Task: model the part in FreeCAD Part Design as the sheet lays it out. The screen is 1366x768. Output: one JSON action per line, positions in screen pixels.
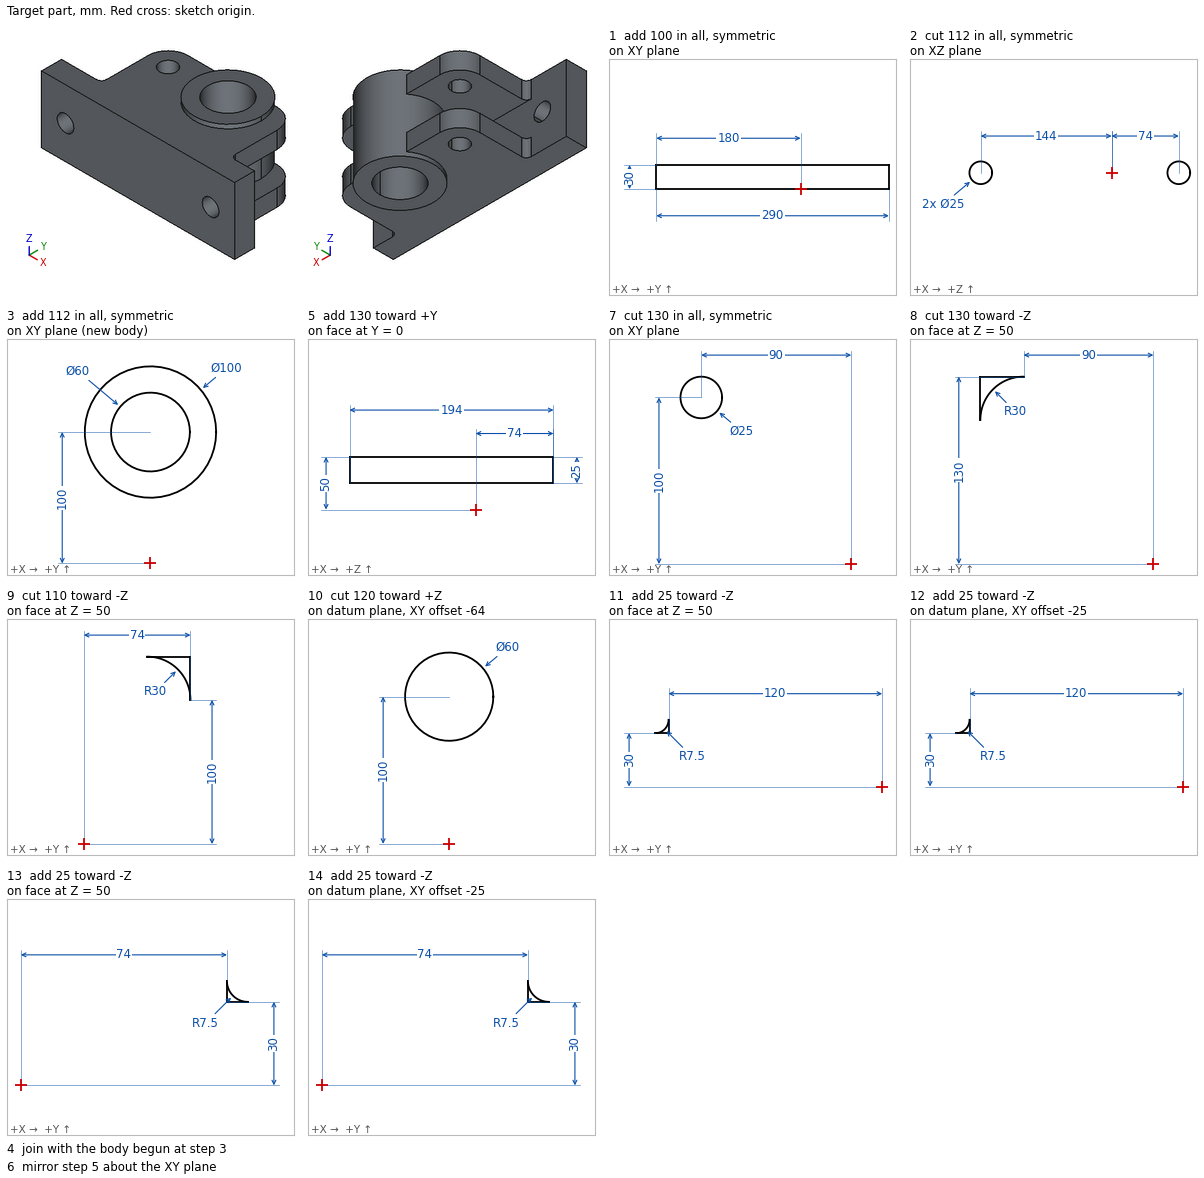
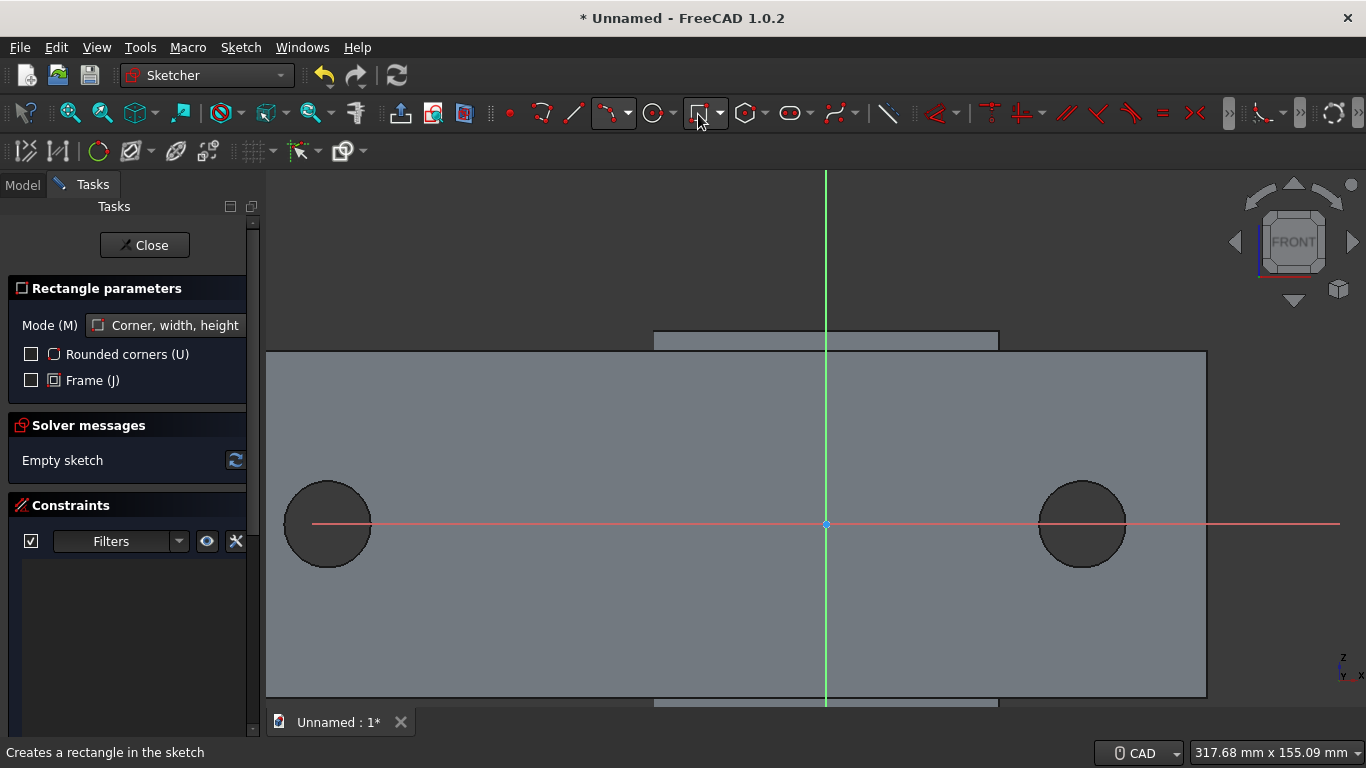
{"action": "left_click", "coordinate": [411, 351]}
{"action": "mouse_move", "coordinate": [1082, 438]}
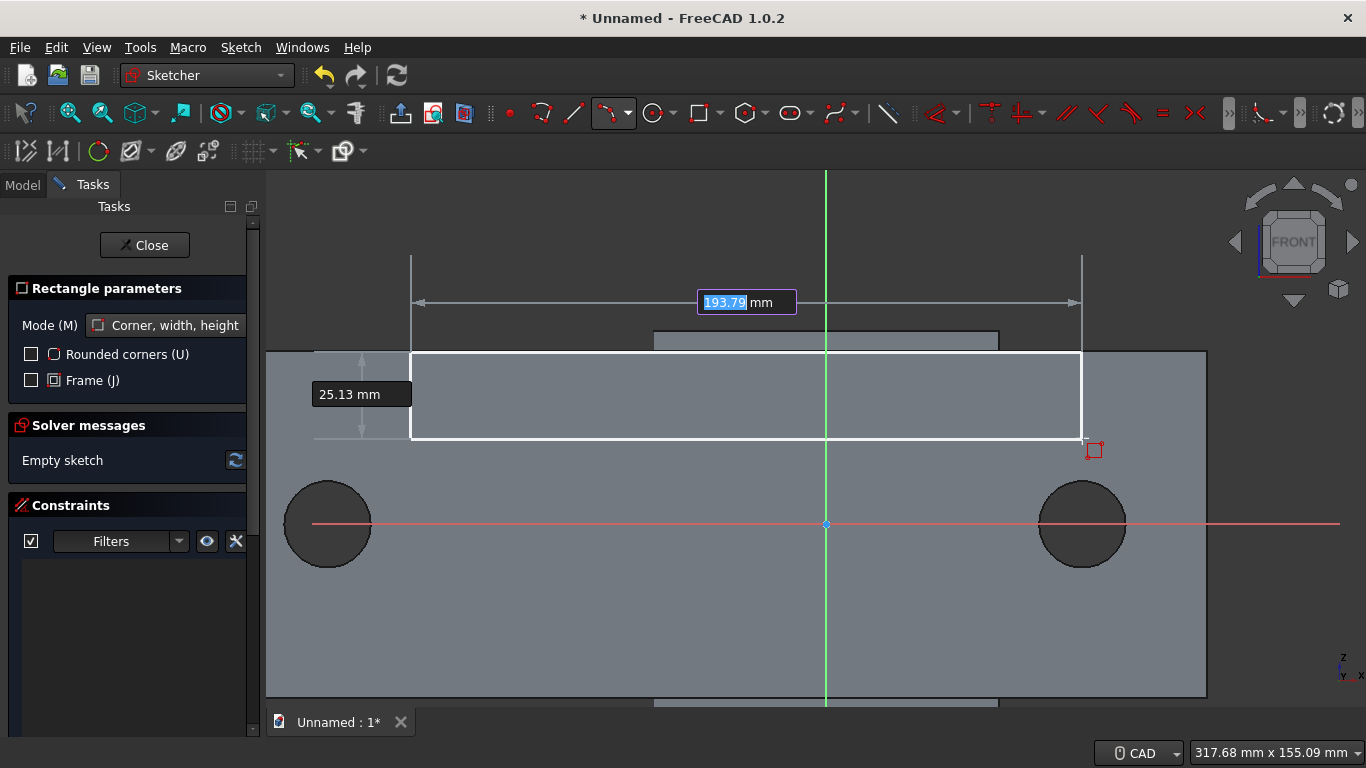
{"action": "type", "text": "194"}
{"action": "key", "text": "Tab"}
{"action": "type", "text": "25"}
{"action": "key", "text": "Return"}
{"action": "key", "text": "Escape"}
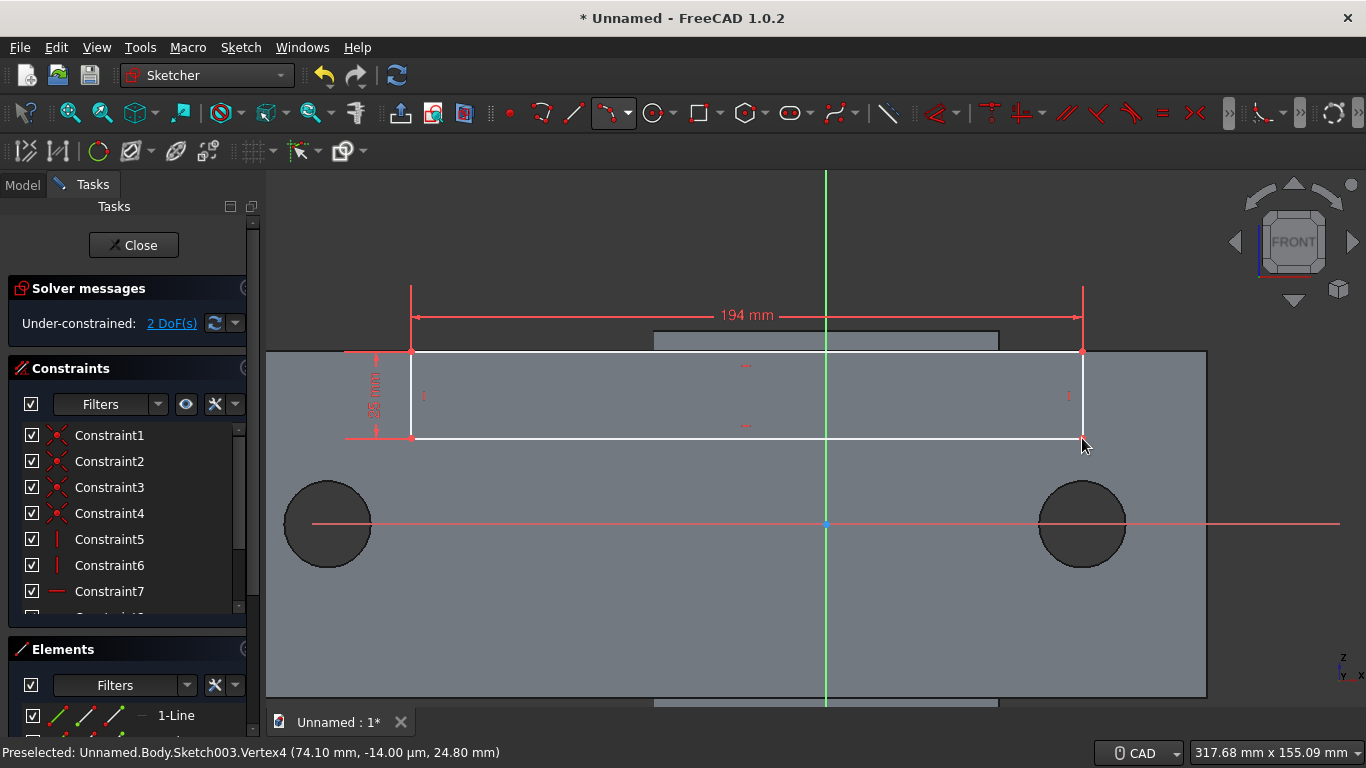
{"action": "left_click", "coordinate": [936, 114]}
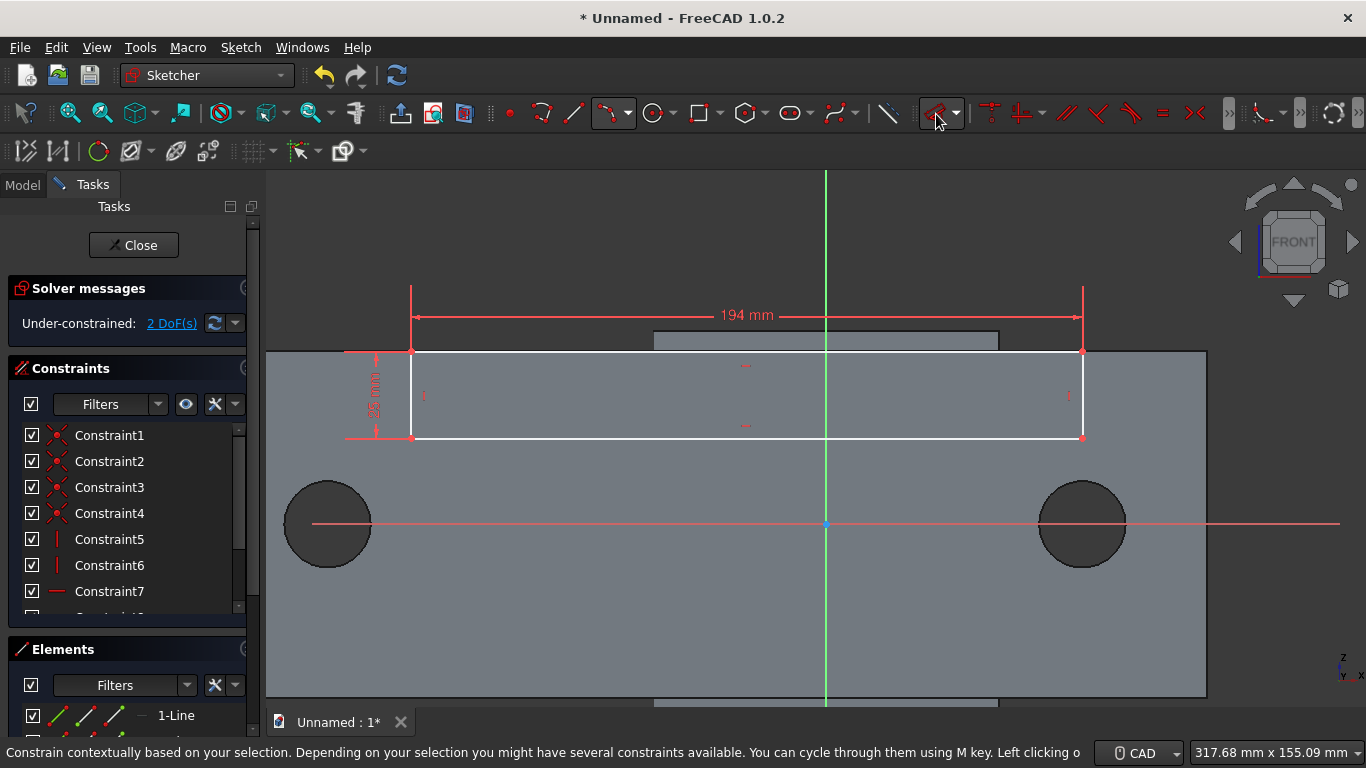
{"action": "left_click", "coordinate": [411, 352]}
{"action": "left_click", "coordinate": [377, 438]}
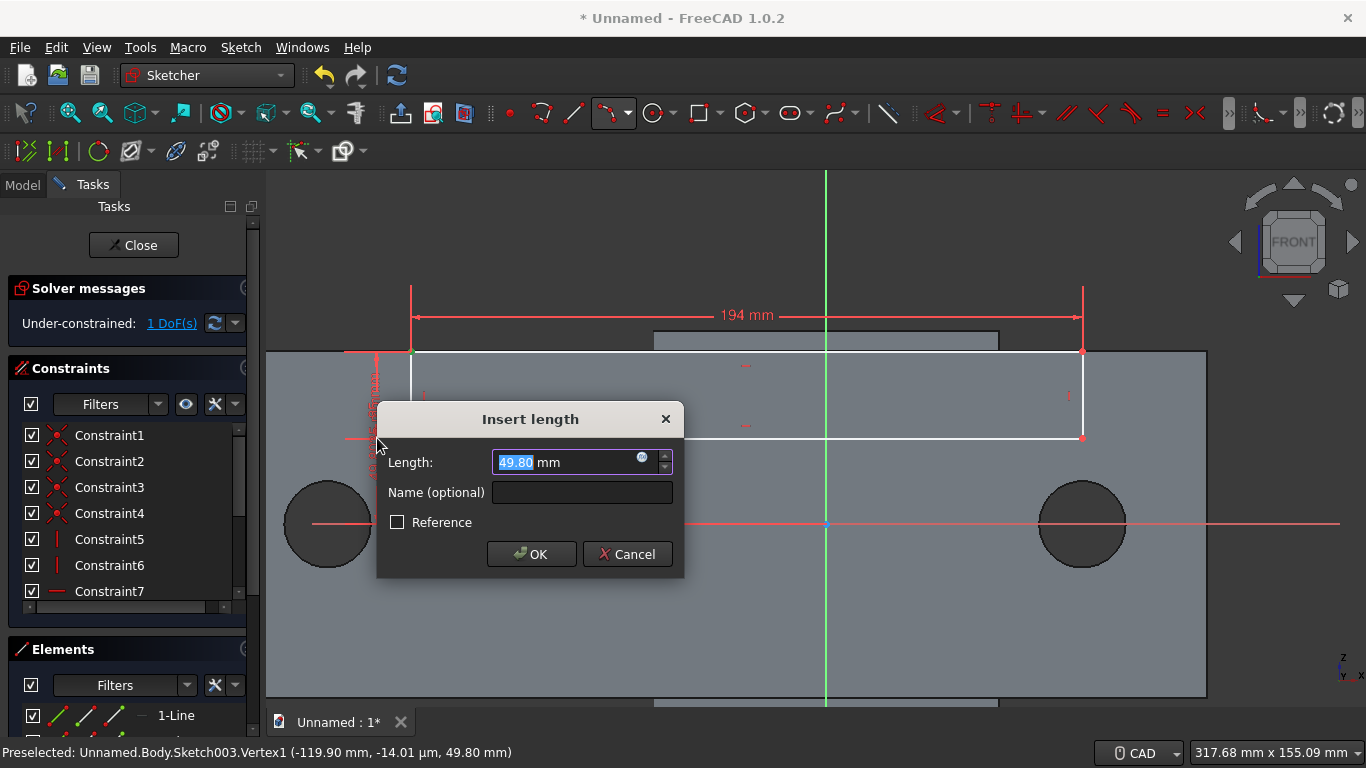
{"action": "type", "text": "50"}
{"action": "key", "text": "Return"}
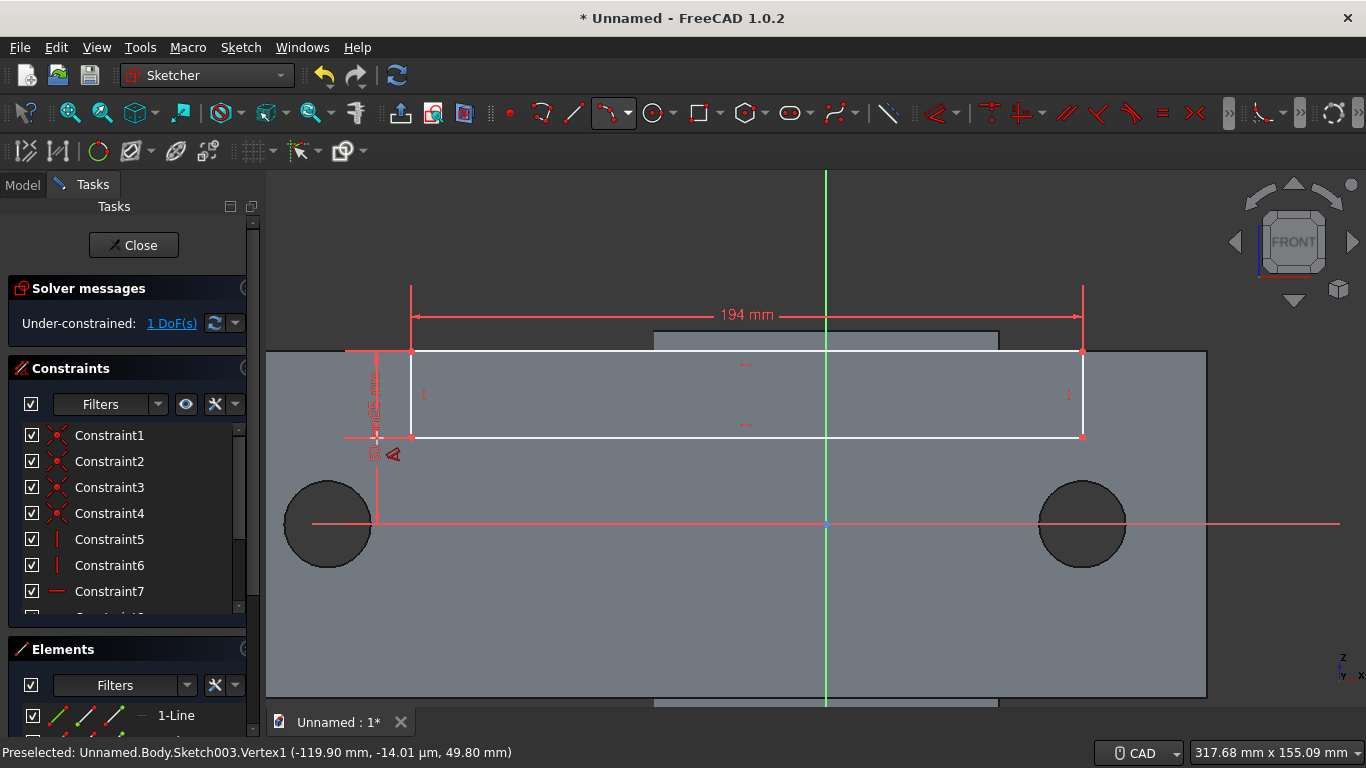
{"action": "left_click", "coordinate": [1083, 438]}
{"action": "left_click", "coordinate": [954, 558]}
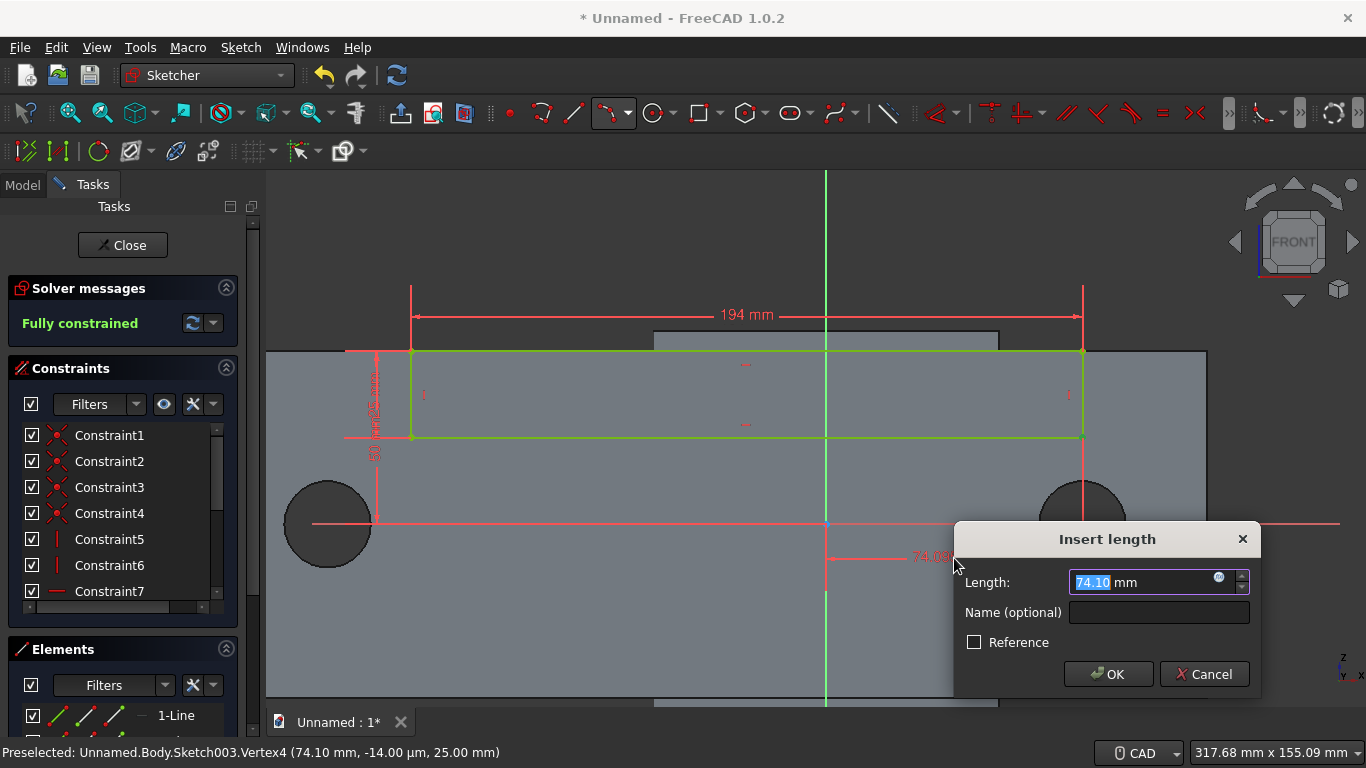
{"action": "type", "text": "74"}
{"action": "key", "text": "Return"}
{"action": "key", "text": "Escape"}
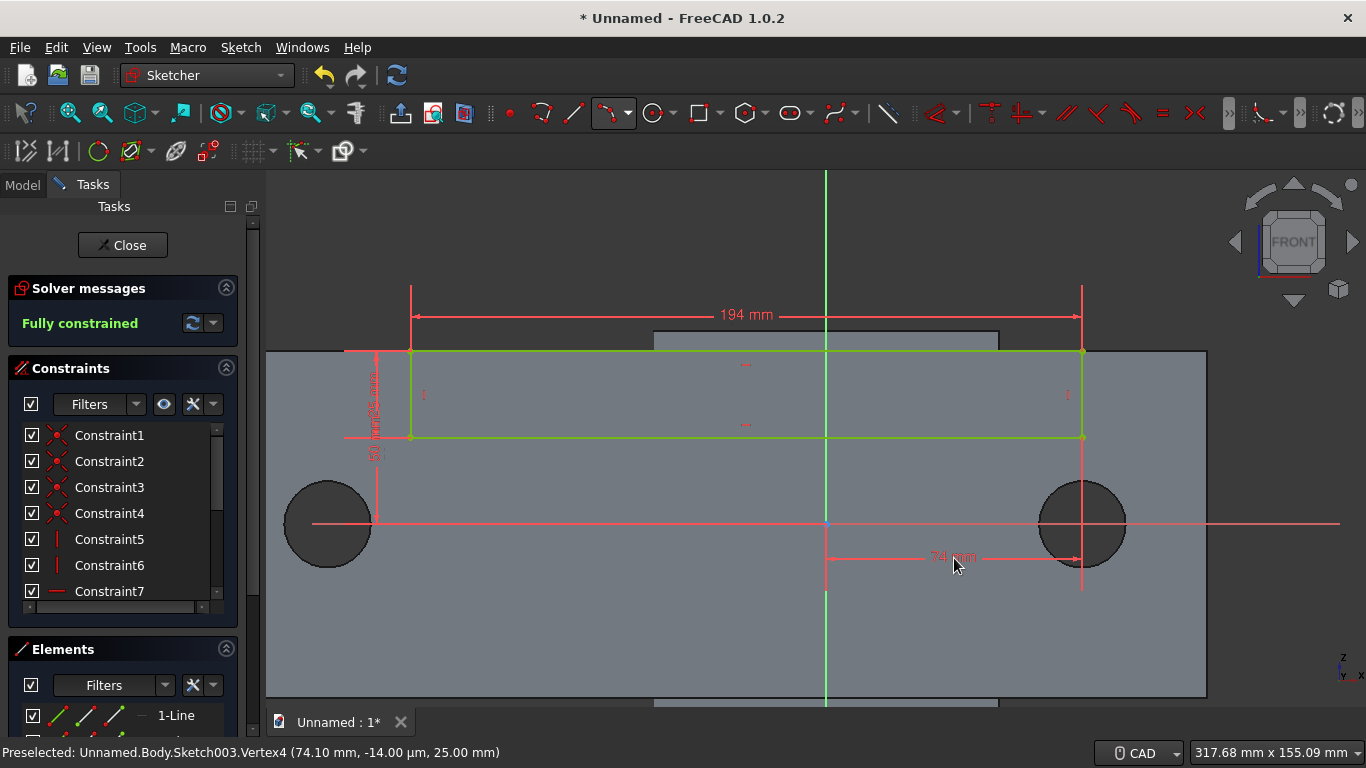
{"action": "left_click", "coordinate": [123, 245]}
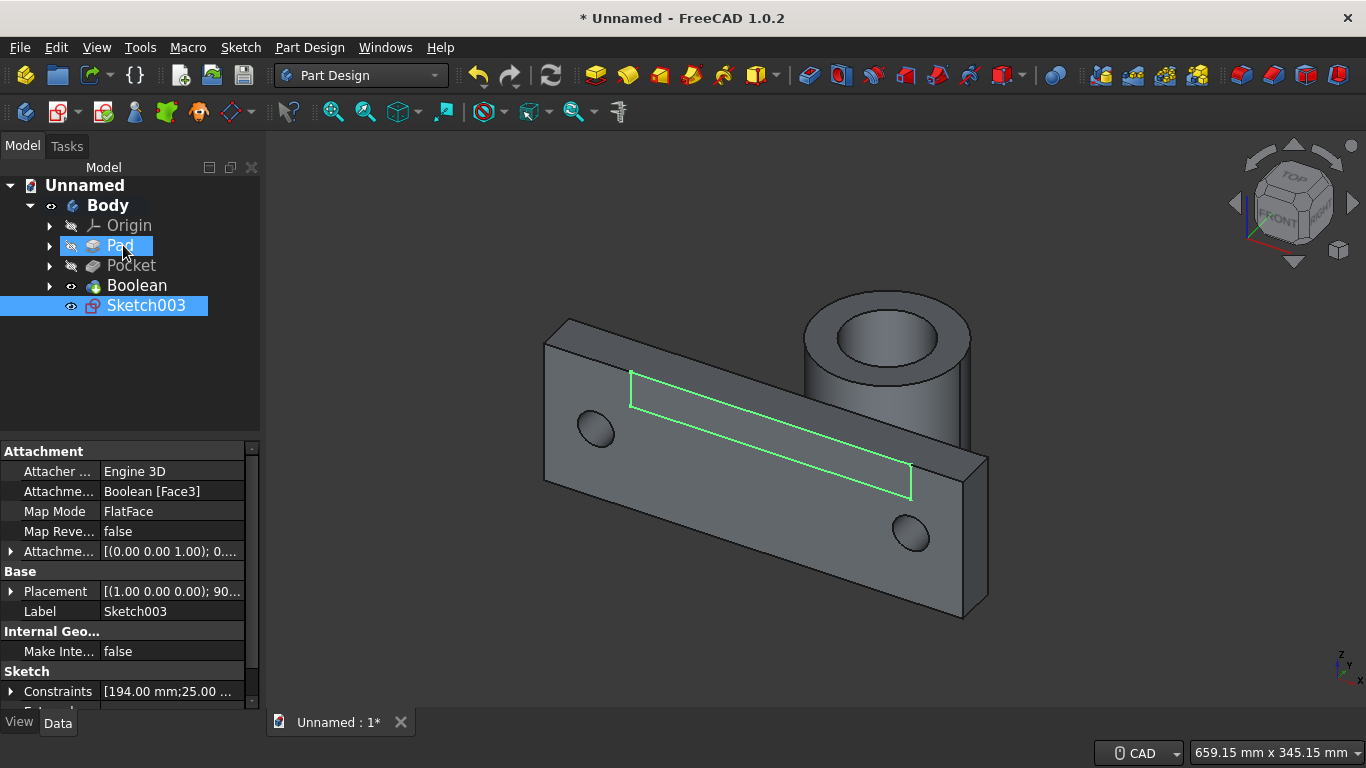
{"action": "left_click", "coordinate": [596, 76]}